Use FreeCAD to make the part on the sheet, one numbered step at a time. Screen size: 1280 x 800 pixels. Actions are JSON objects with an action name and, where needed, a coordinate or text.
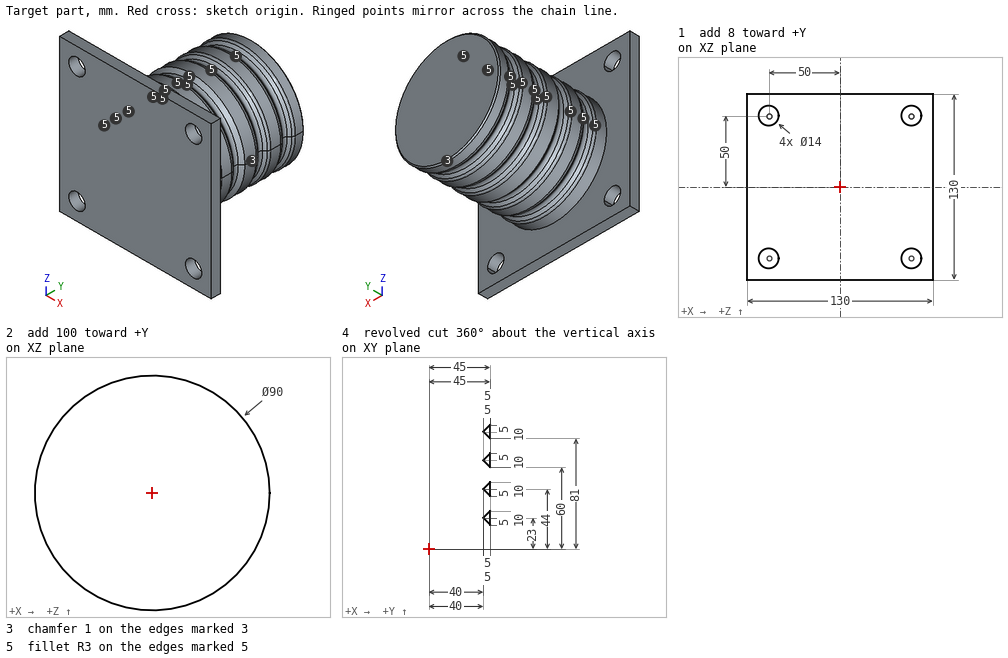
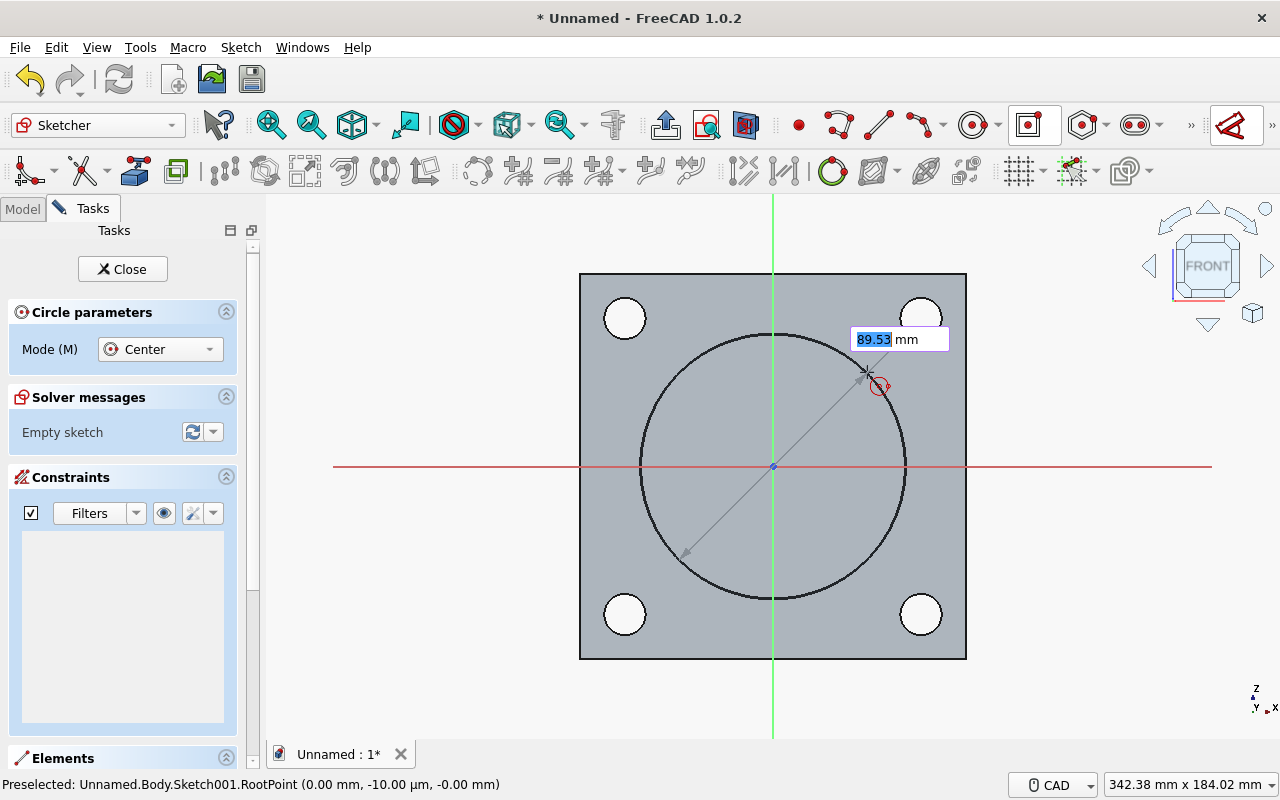
{"action": "type", "text": "90"}
{"action": "key", "text": "Return"}
{"action": "key", "text": "Escape"}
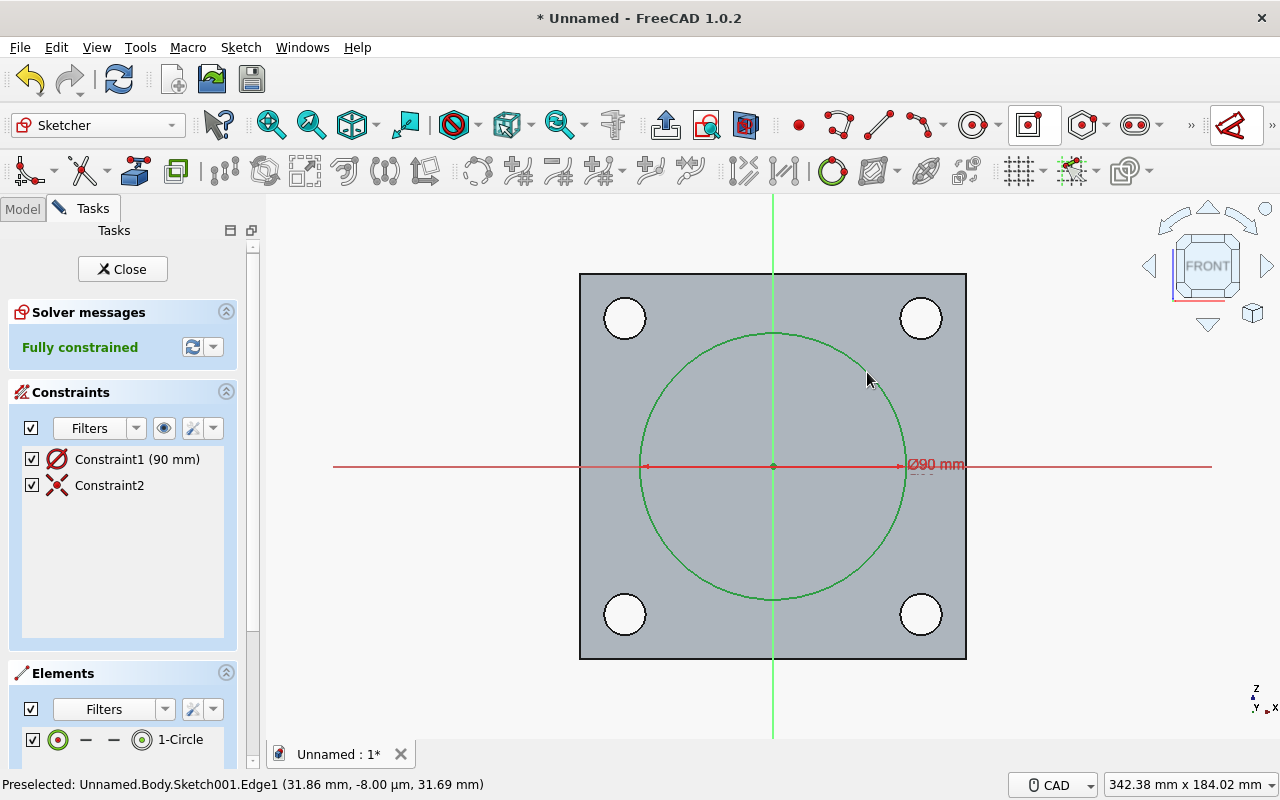
{"action": "left_click", "coordinate": [123, 269]}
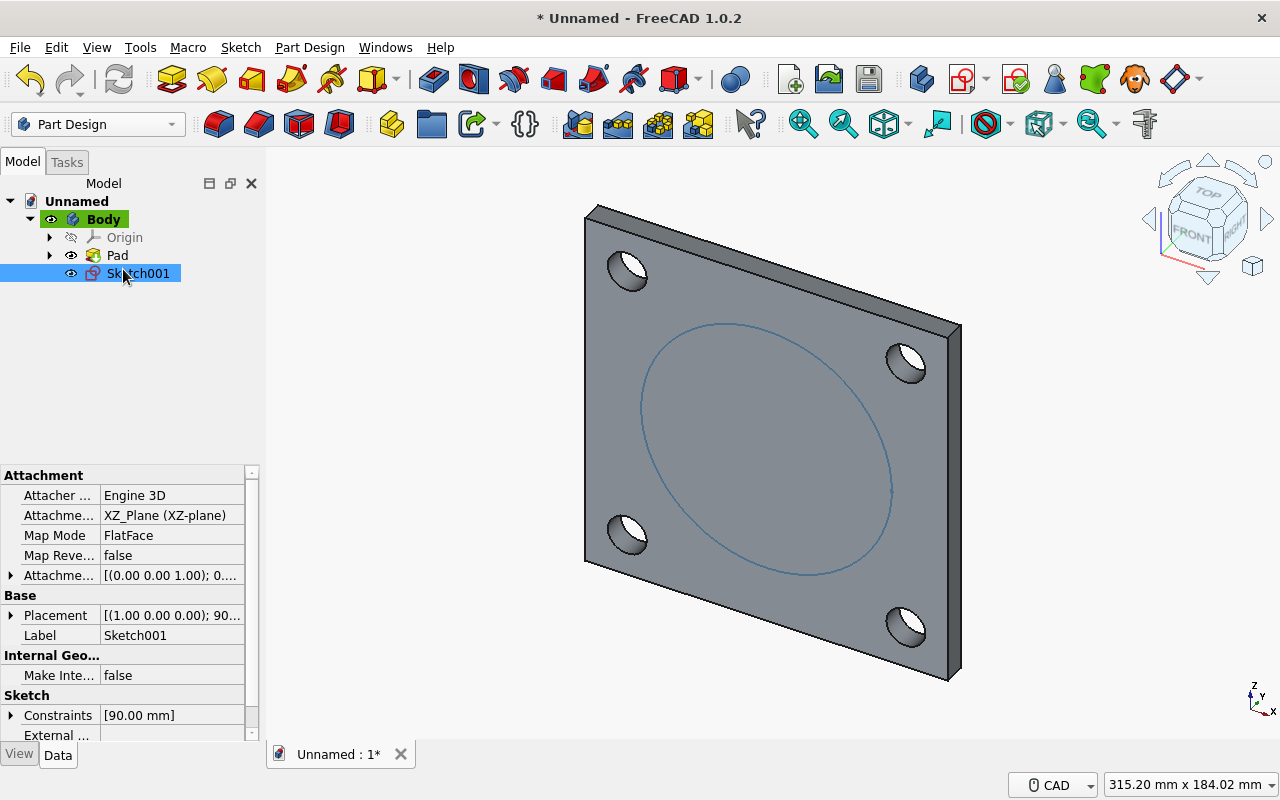
{"action": "left_click", "coordinate": [172, 80]}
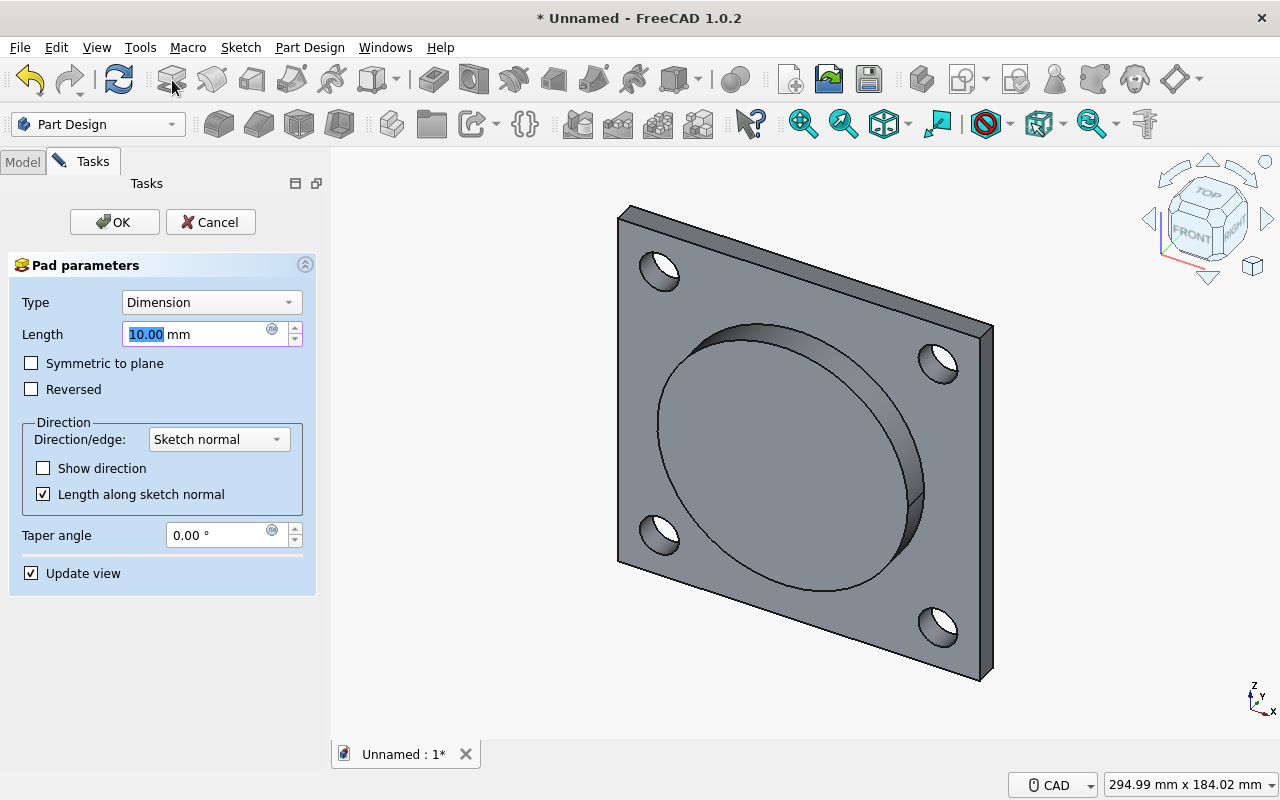
{"action": "type", "text": "100"}
{"action": "key", "text": "Tab"}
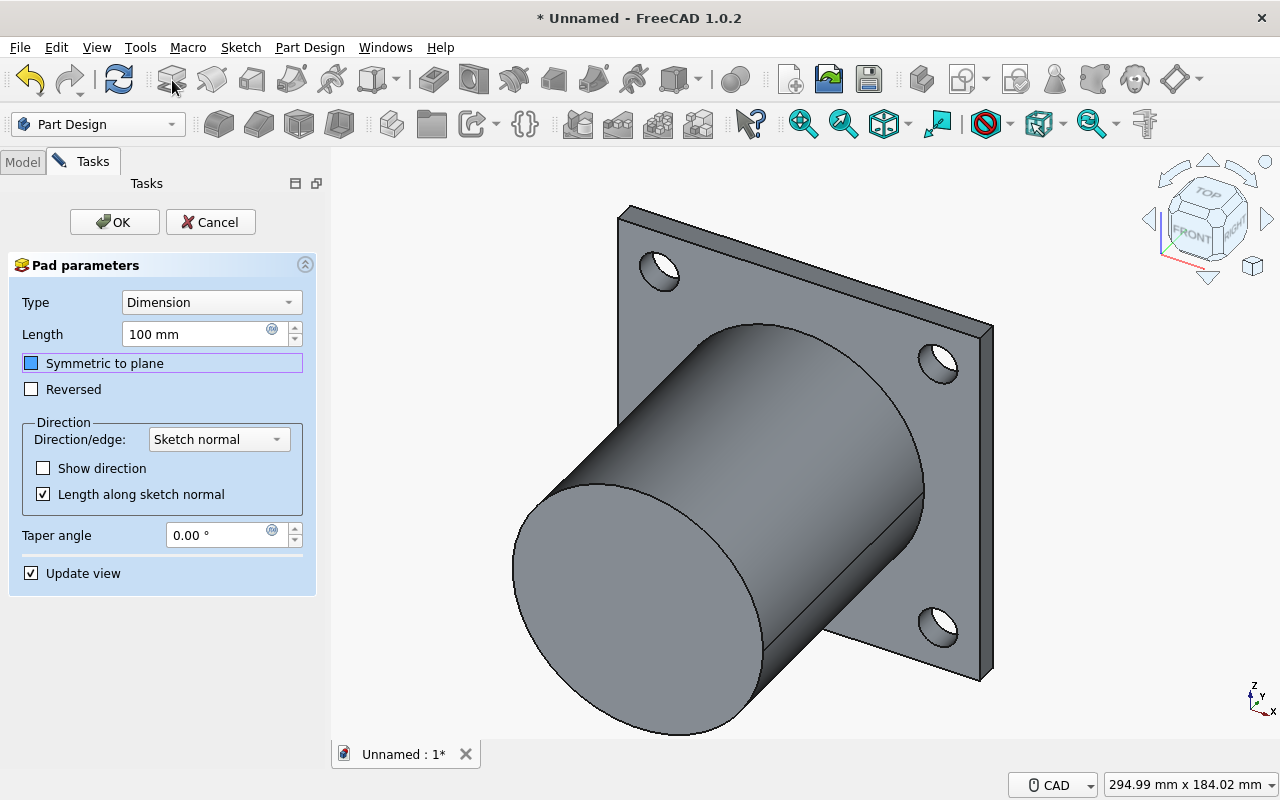
{"action": "left_click", "coordinate": [30, 389]}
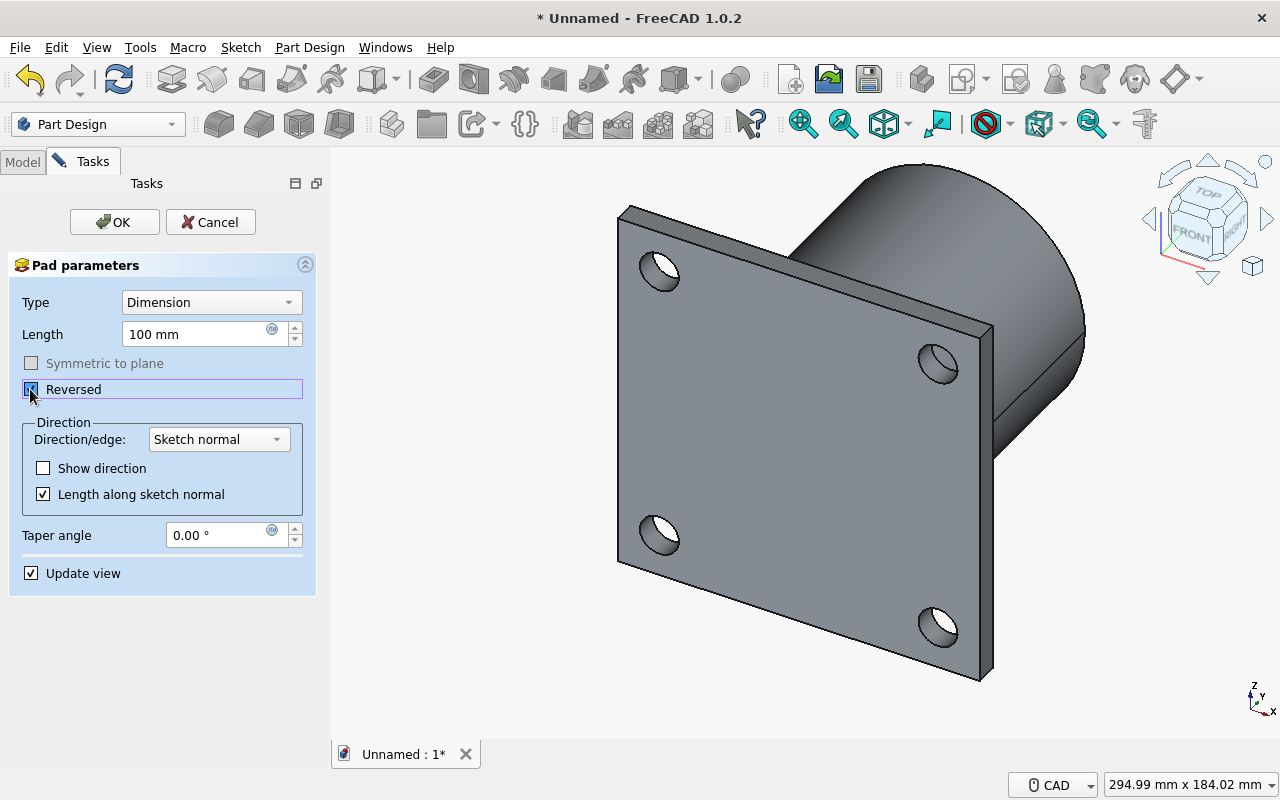
{"action": "left_click", "coordinate": [115, 222]}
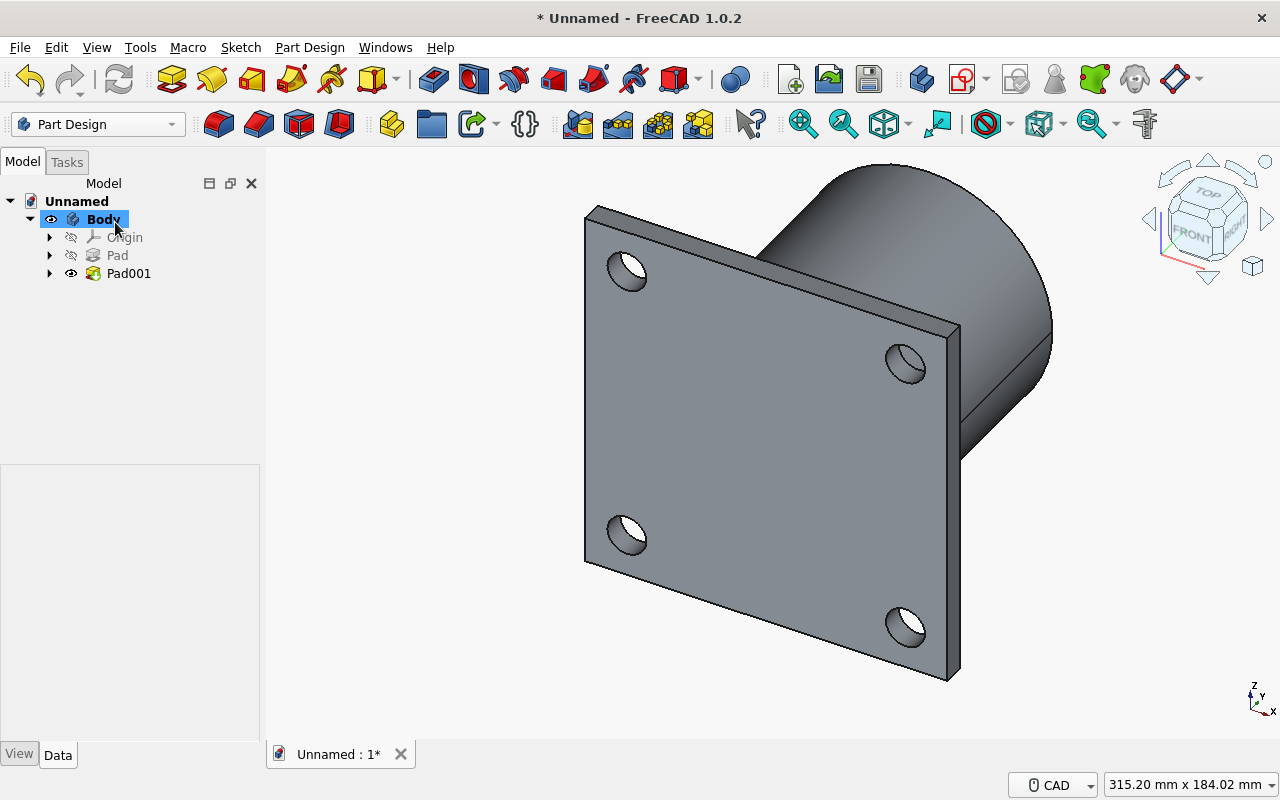
{"action": "key", "text": "v f"}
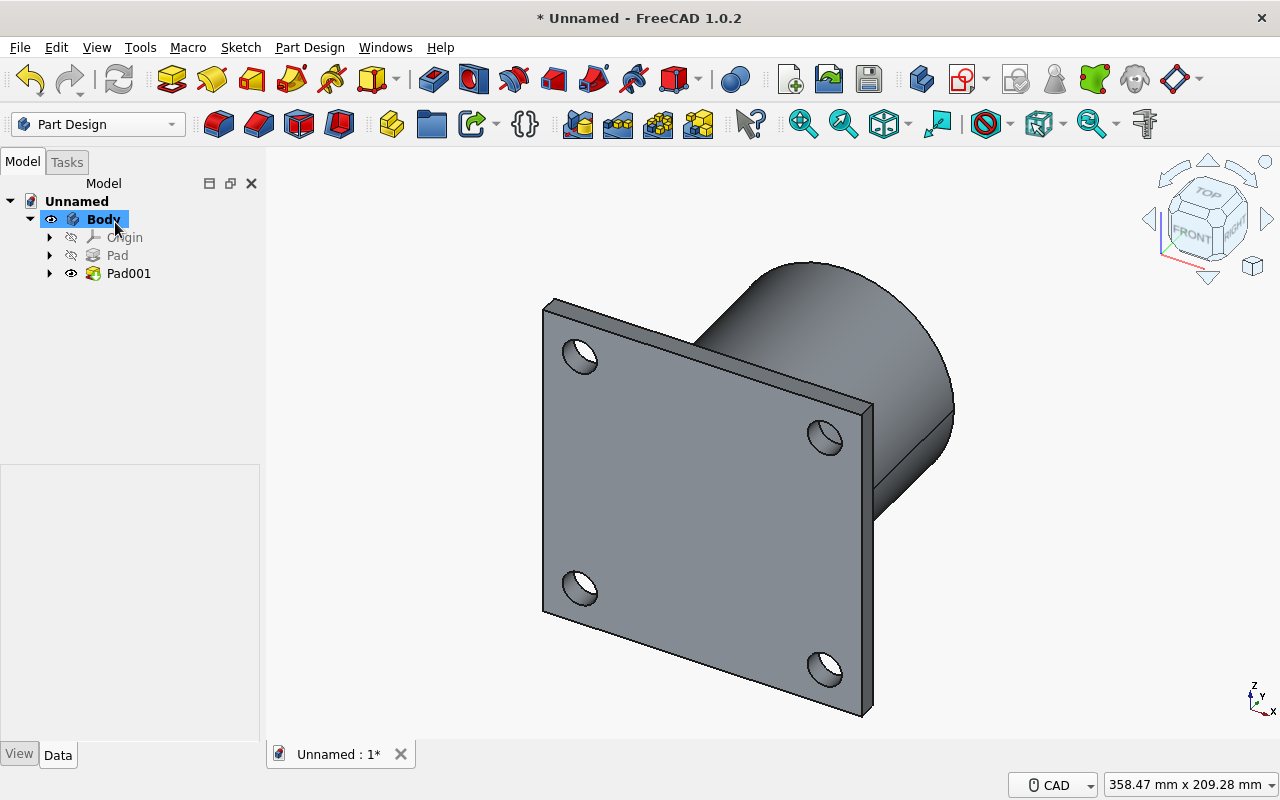
{"action": "key", "text": "0"}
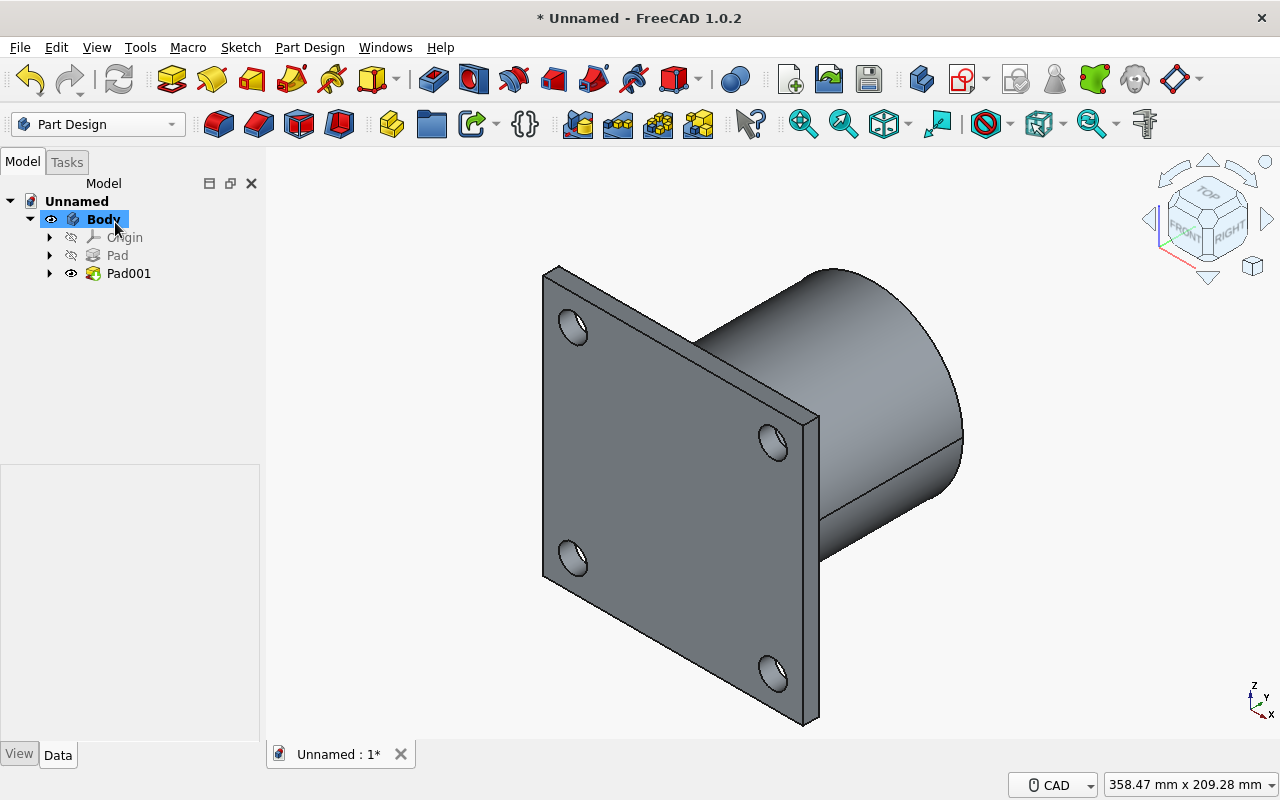
{"action": "left_click", "coordinate": [845, 269]}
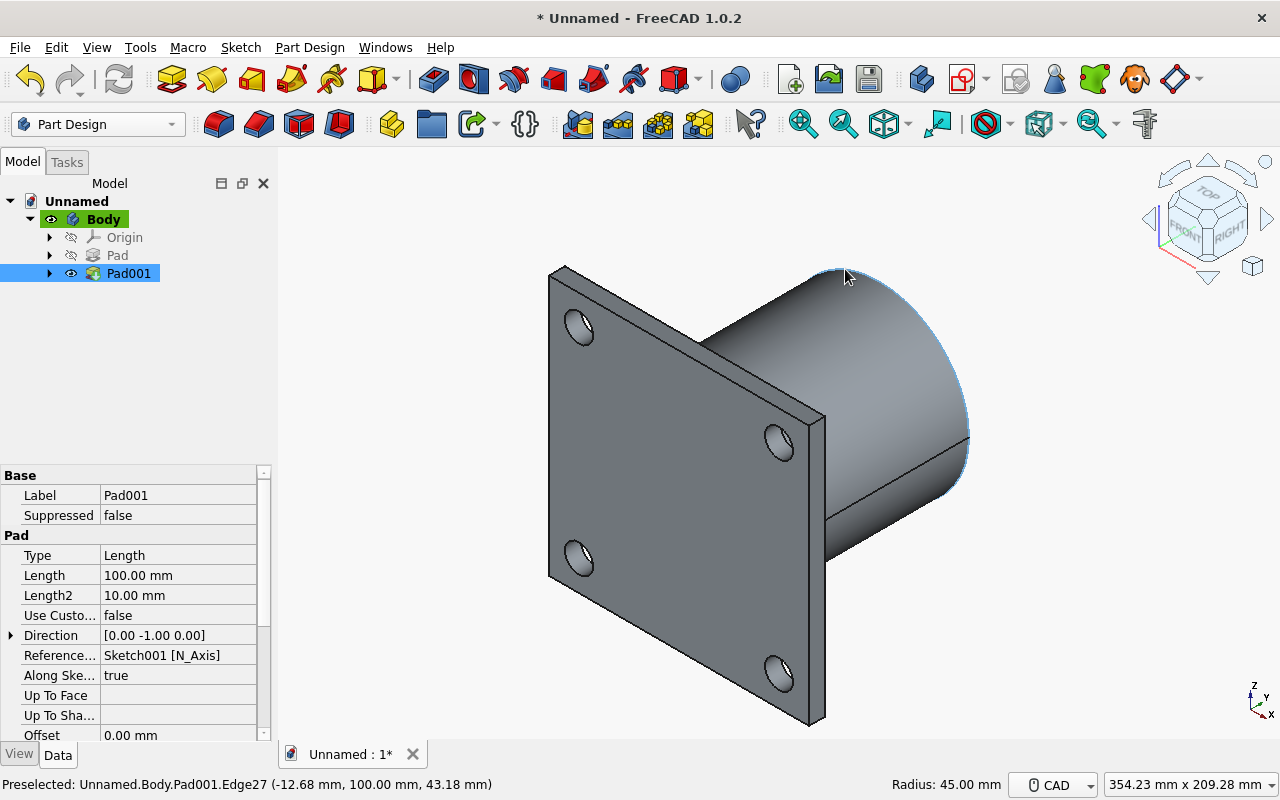
{"action": "left_click", "coordinate": [260, 124]}